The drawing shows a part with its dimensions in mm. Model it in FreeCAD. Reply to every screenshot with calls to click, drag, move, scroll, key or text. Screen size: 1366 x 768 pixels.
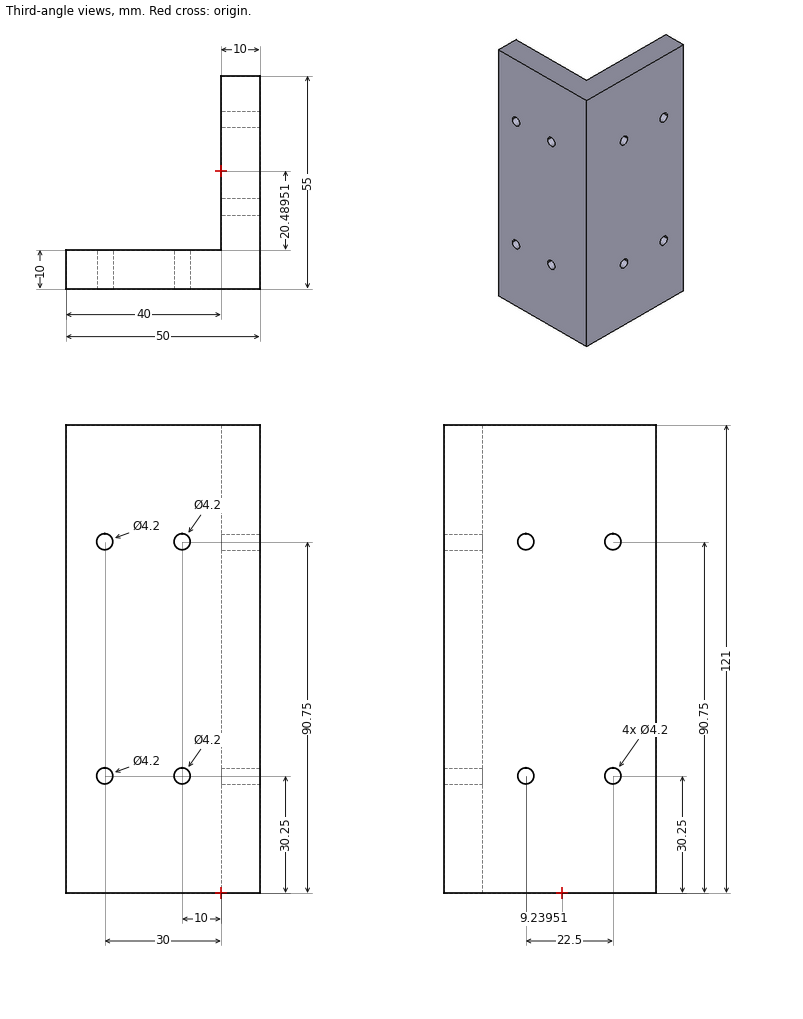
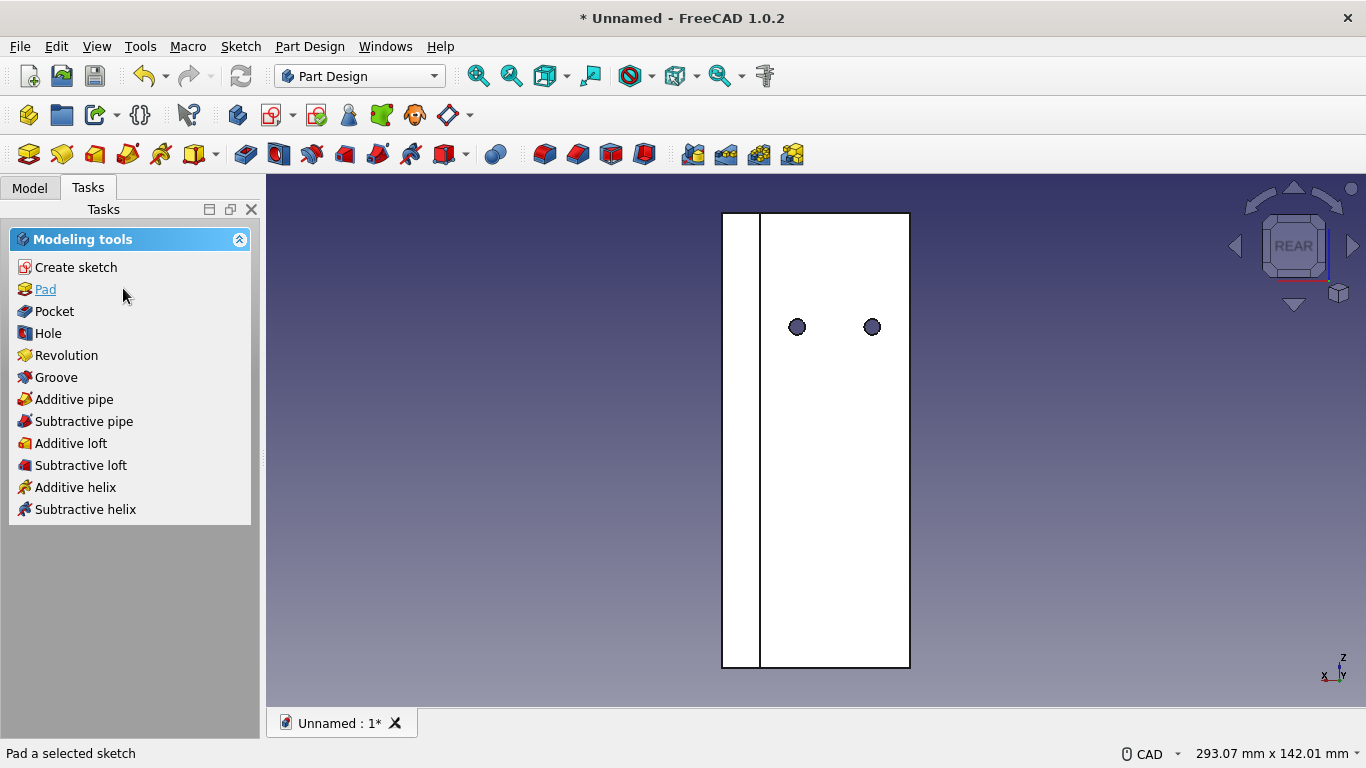
click(246, 154)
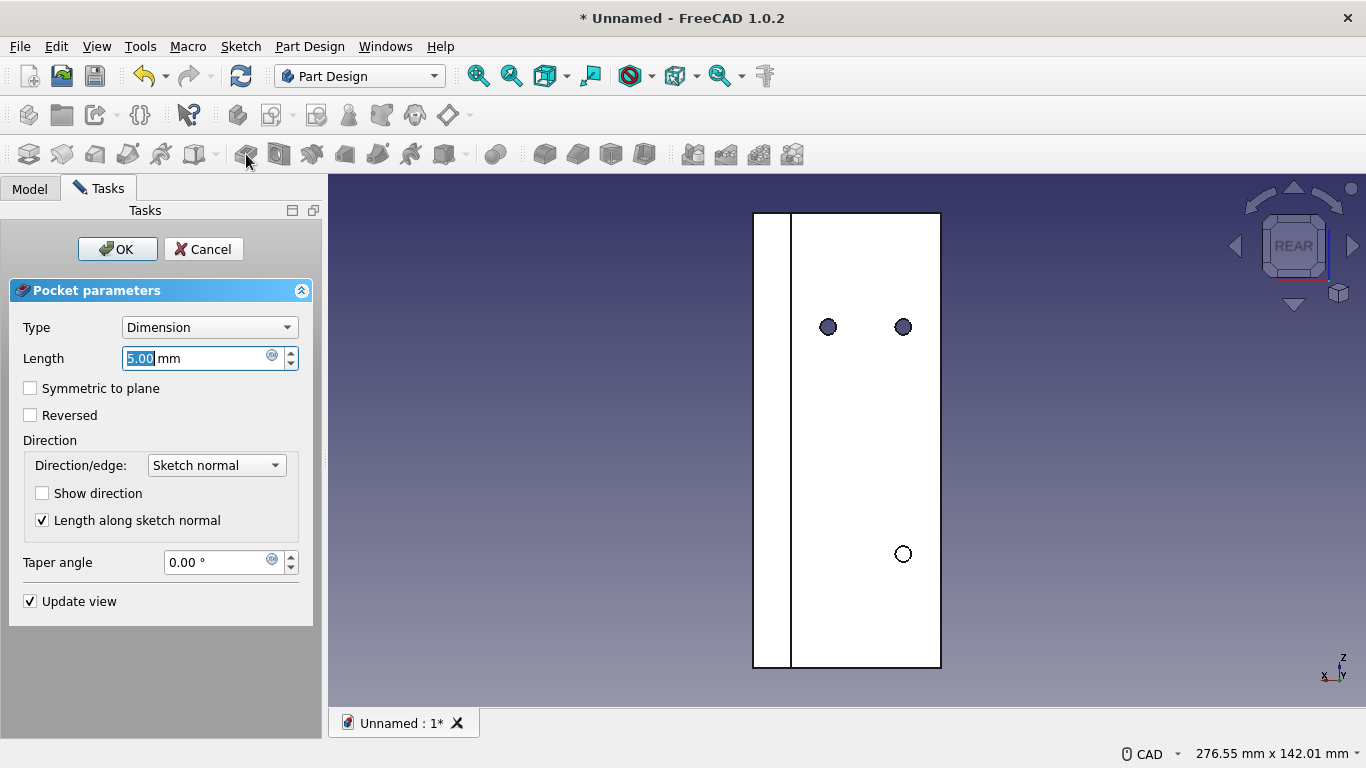
click(210, 328)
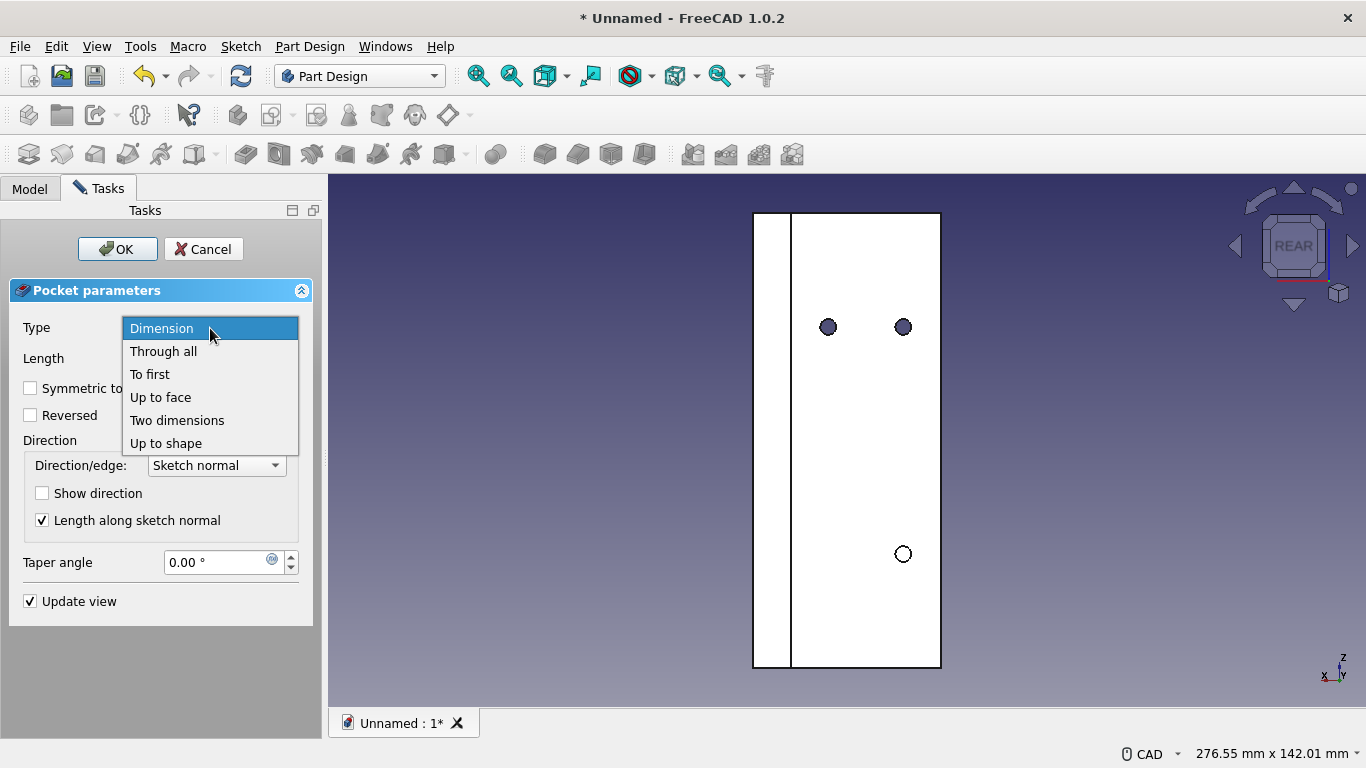
click(208, 374)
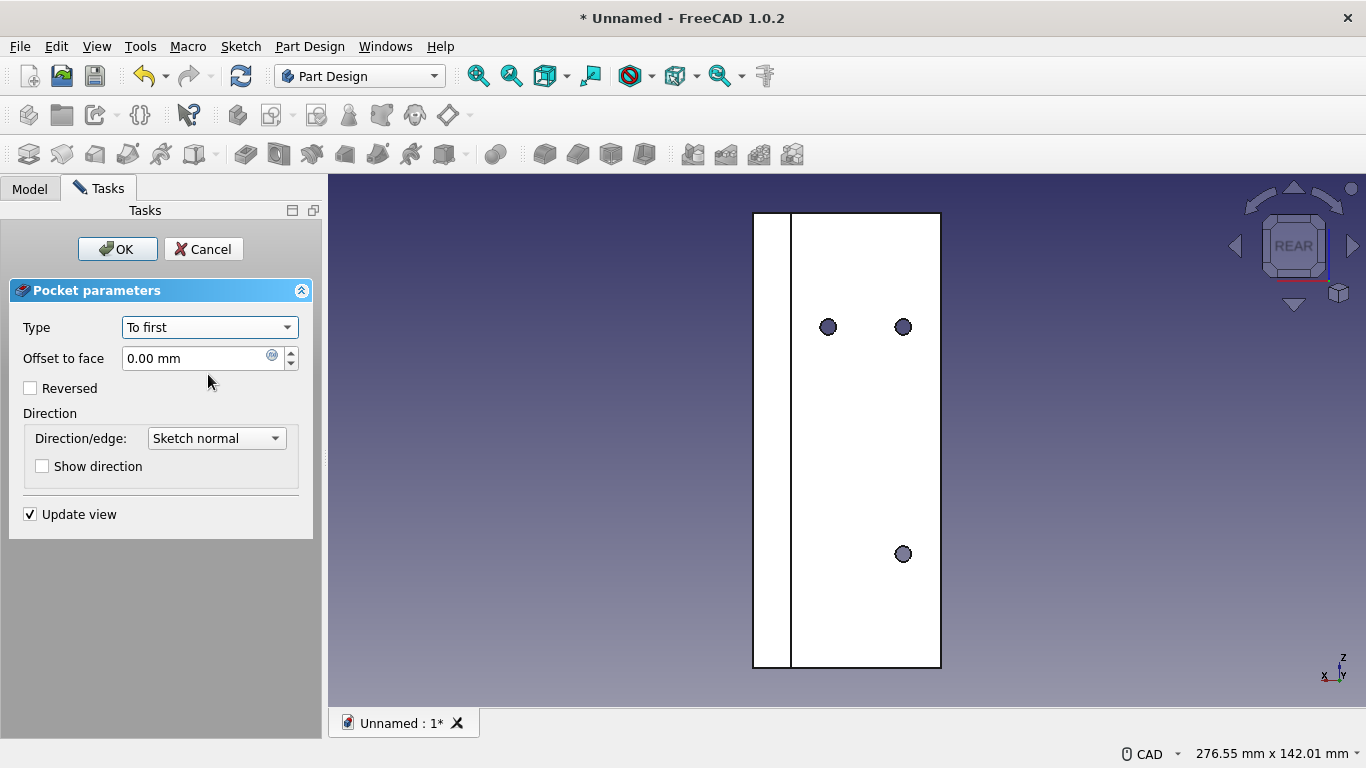
click(118, 249)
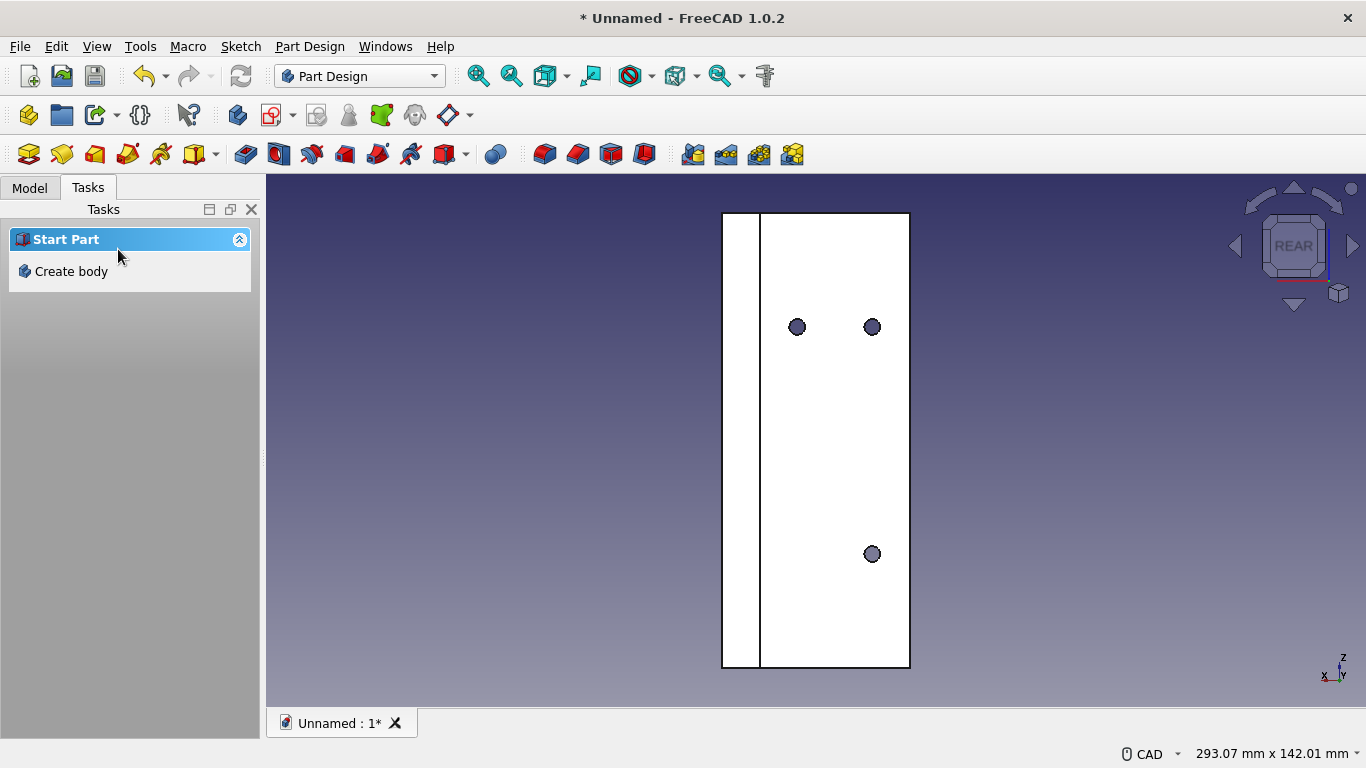
click(835, 439)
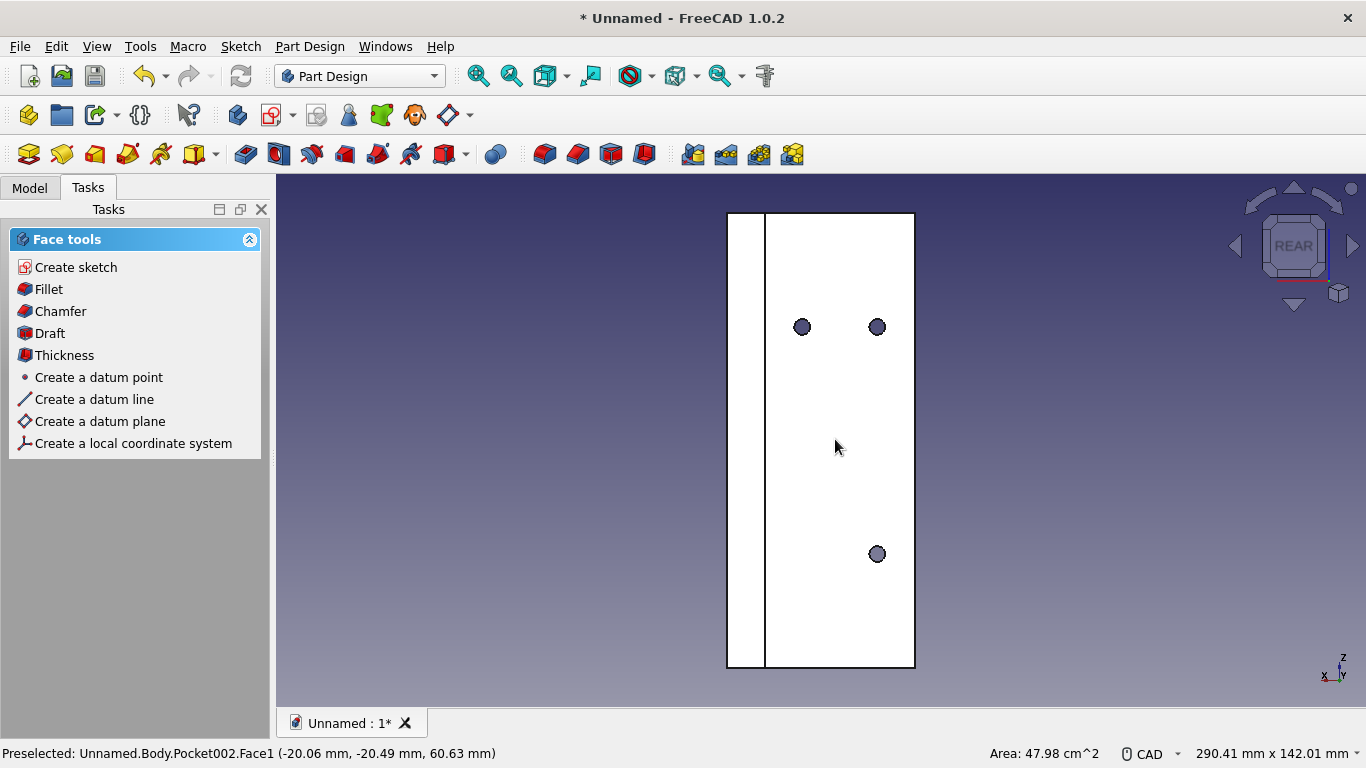
click(270, 116)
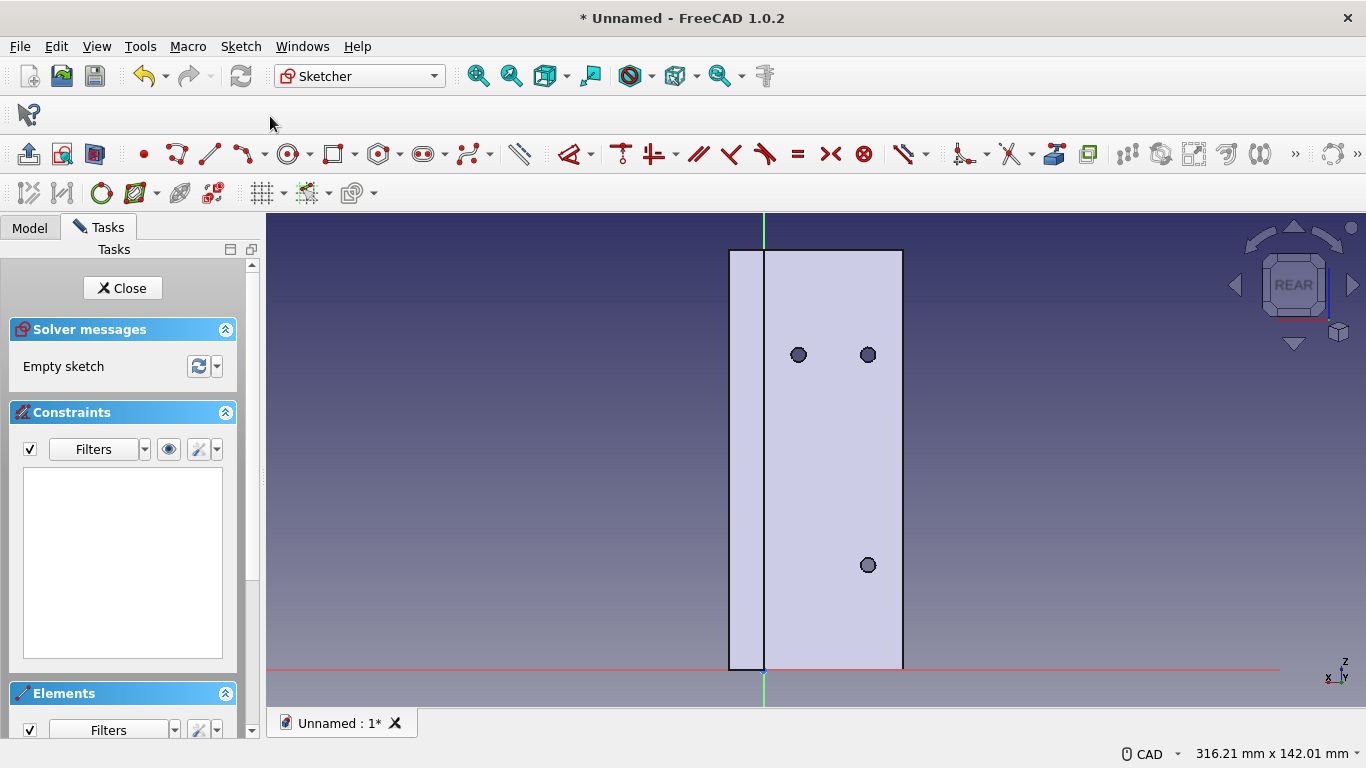
scroll(801, 571, up, 15)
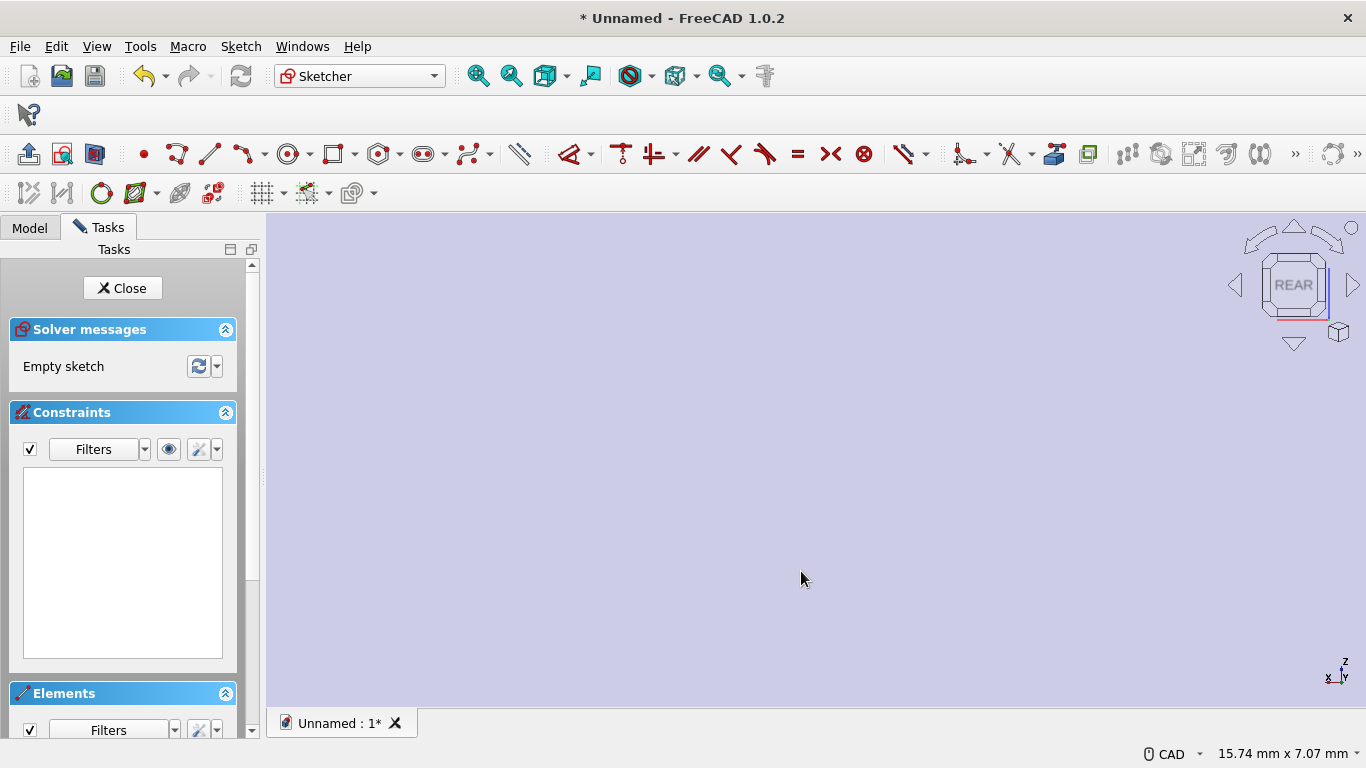
key(g)
key(c)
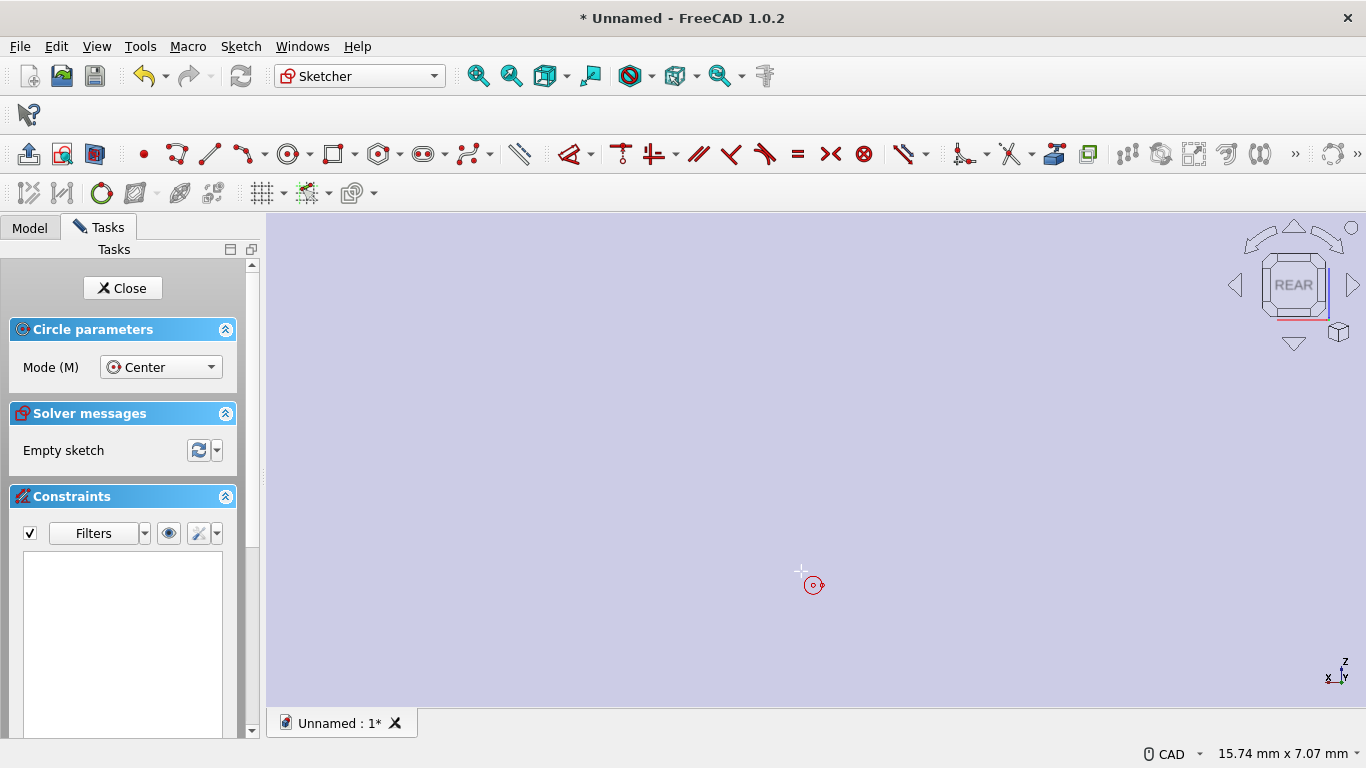
click(744, 441)
move(847, 338)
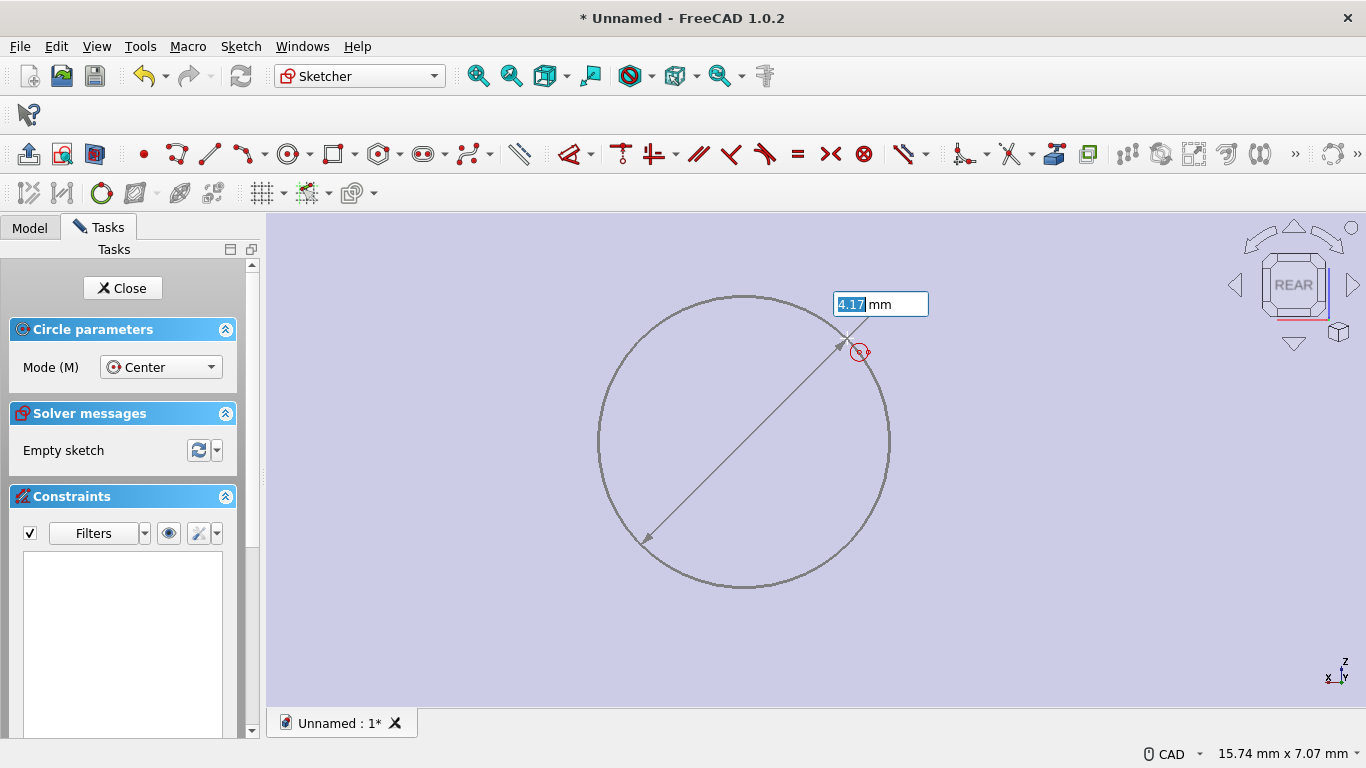
text(4.2)
key(Return)
key(Escape)